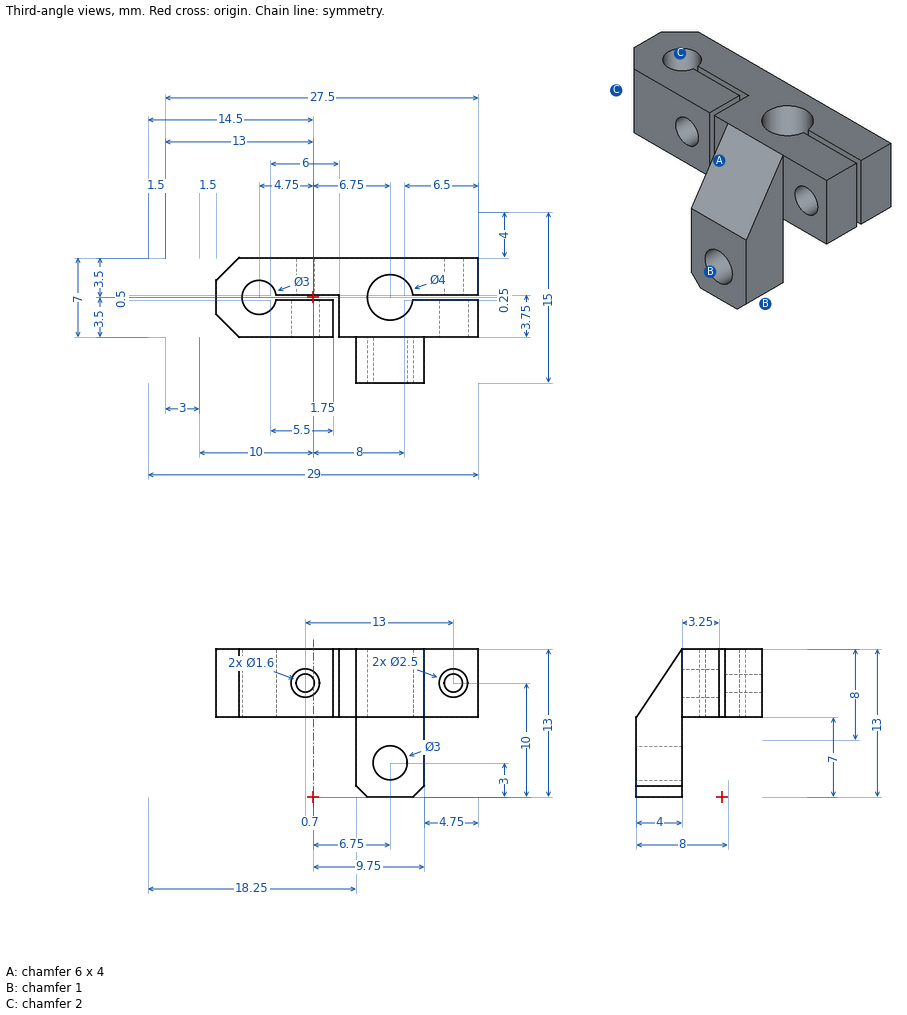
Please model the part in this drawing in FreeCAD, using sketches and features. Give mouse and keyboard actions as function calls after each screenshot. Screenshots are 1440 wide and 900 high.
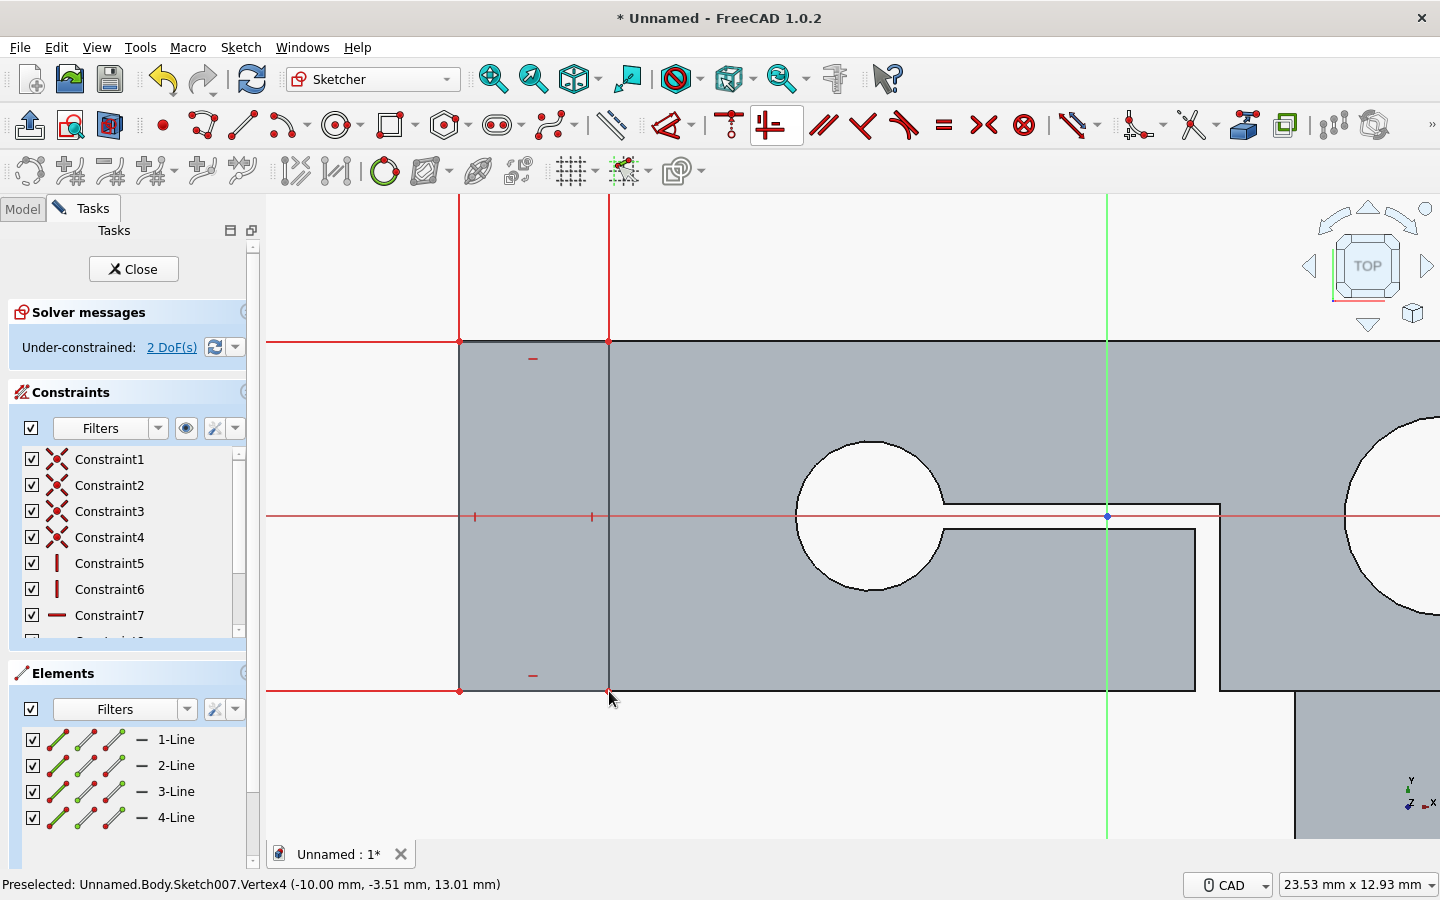
click(666, 126)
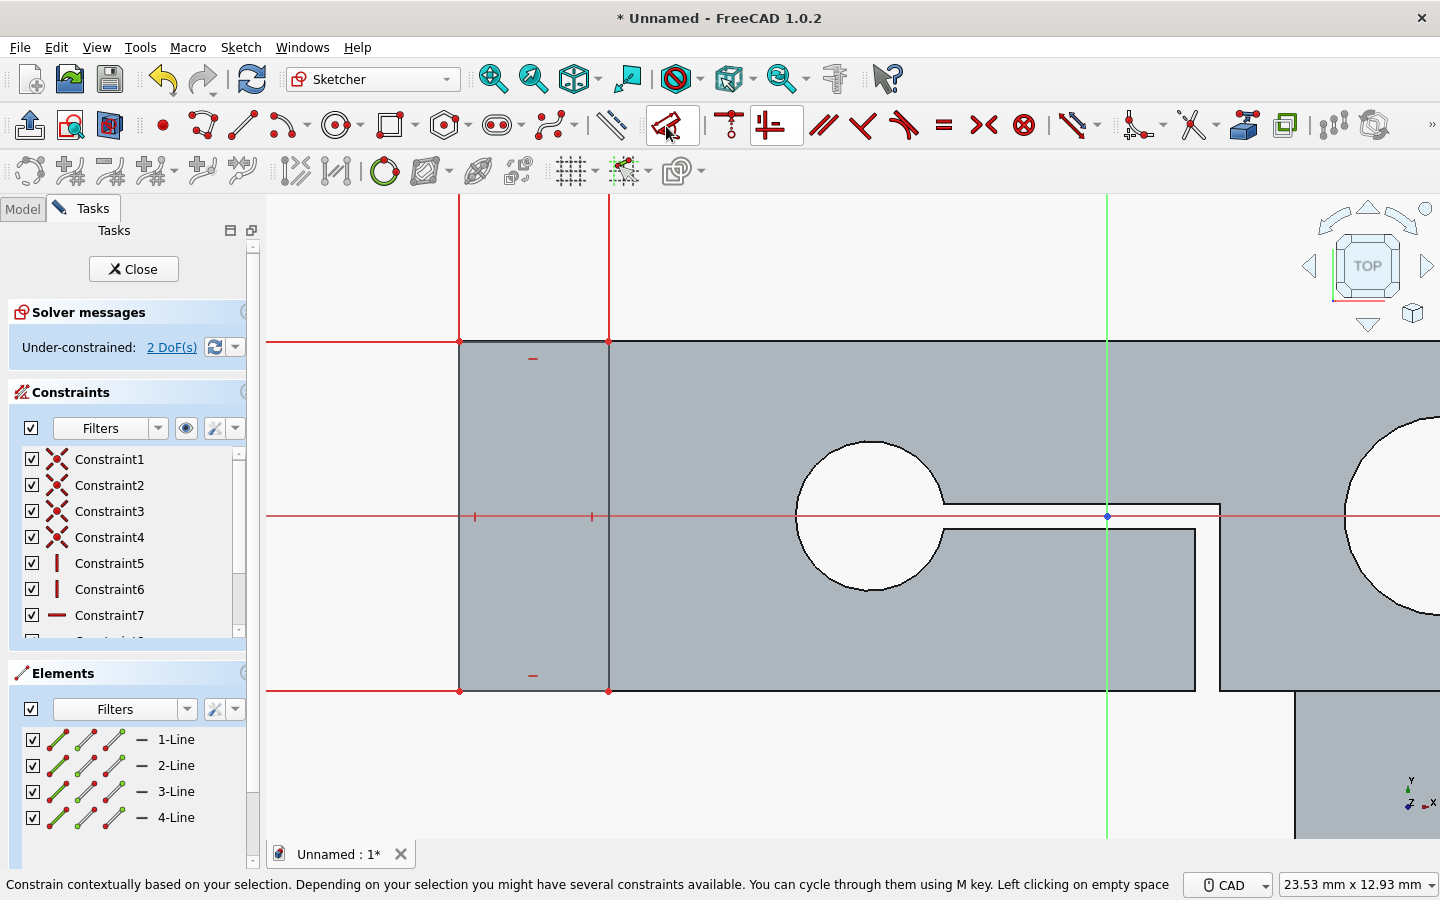
click(459, 342)
click(783, 308)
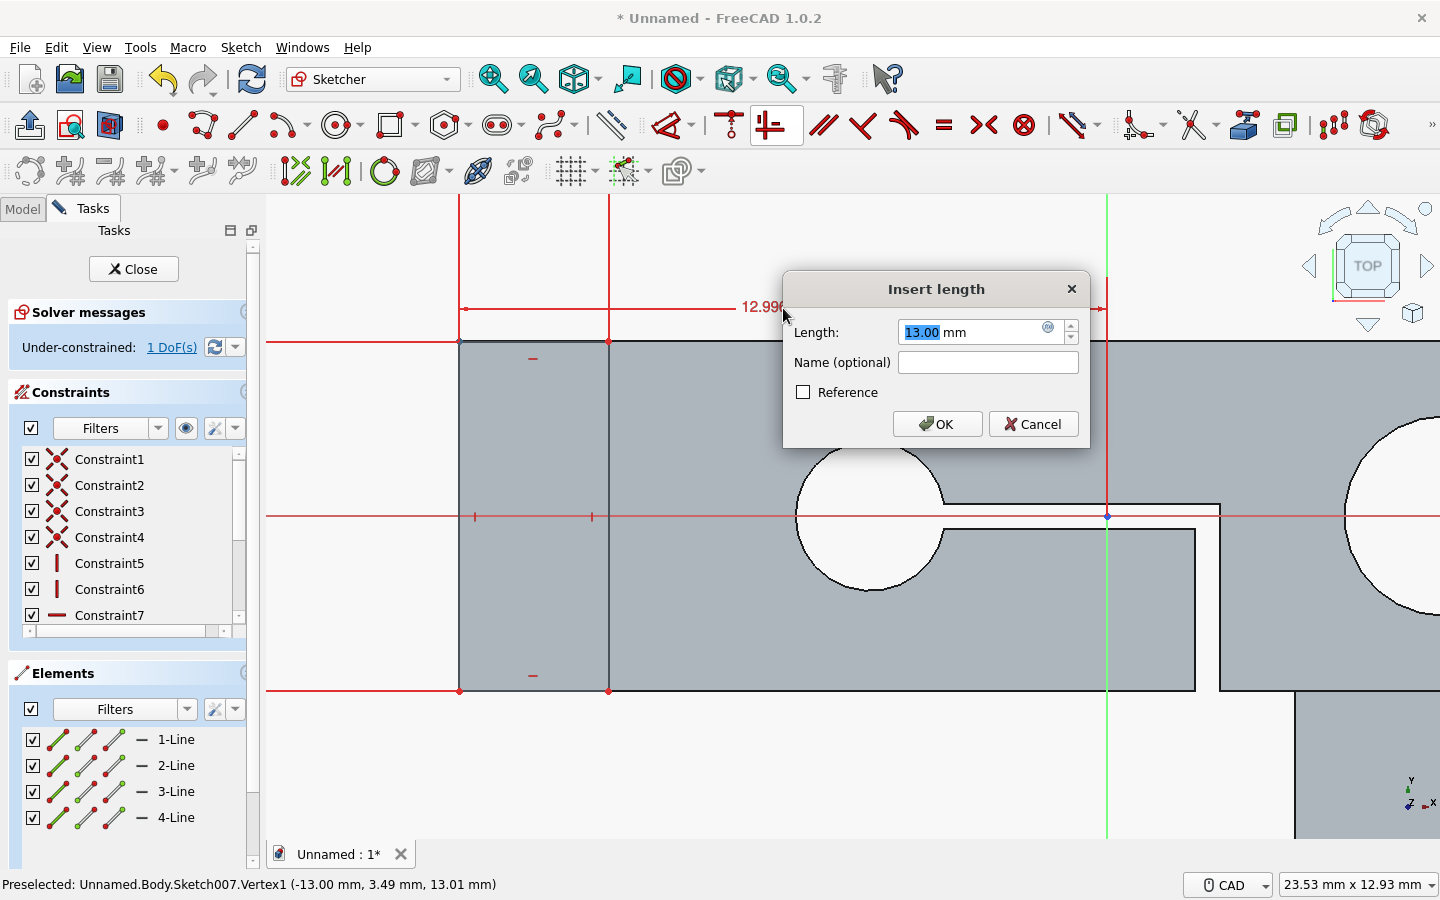
text(13)
key(Return)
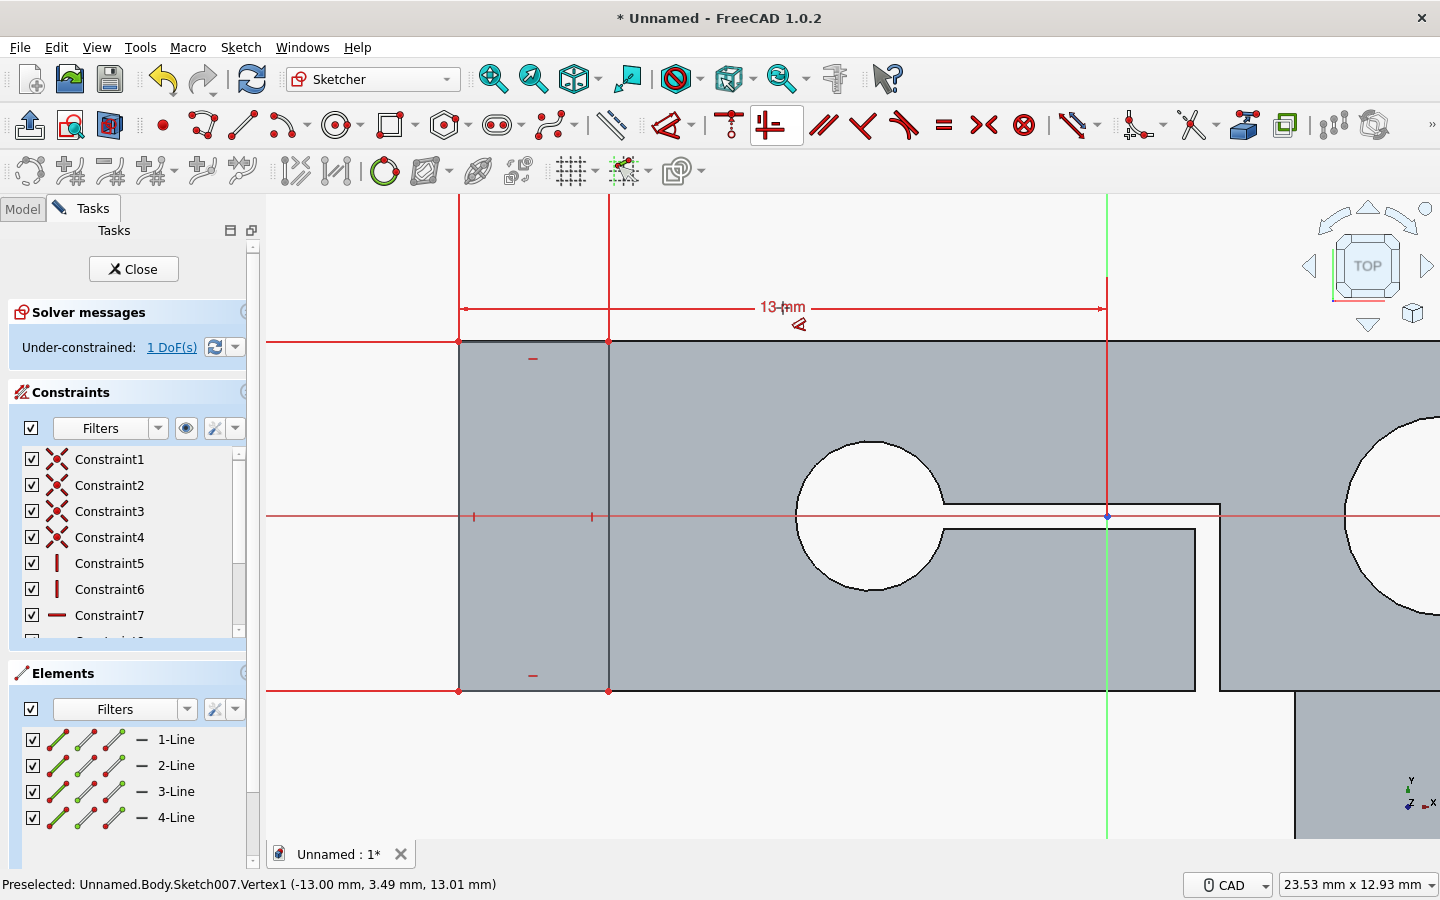
click(459, 342)
click(1141, 429)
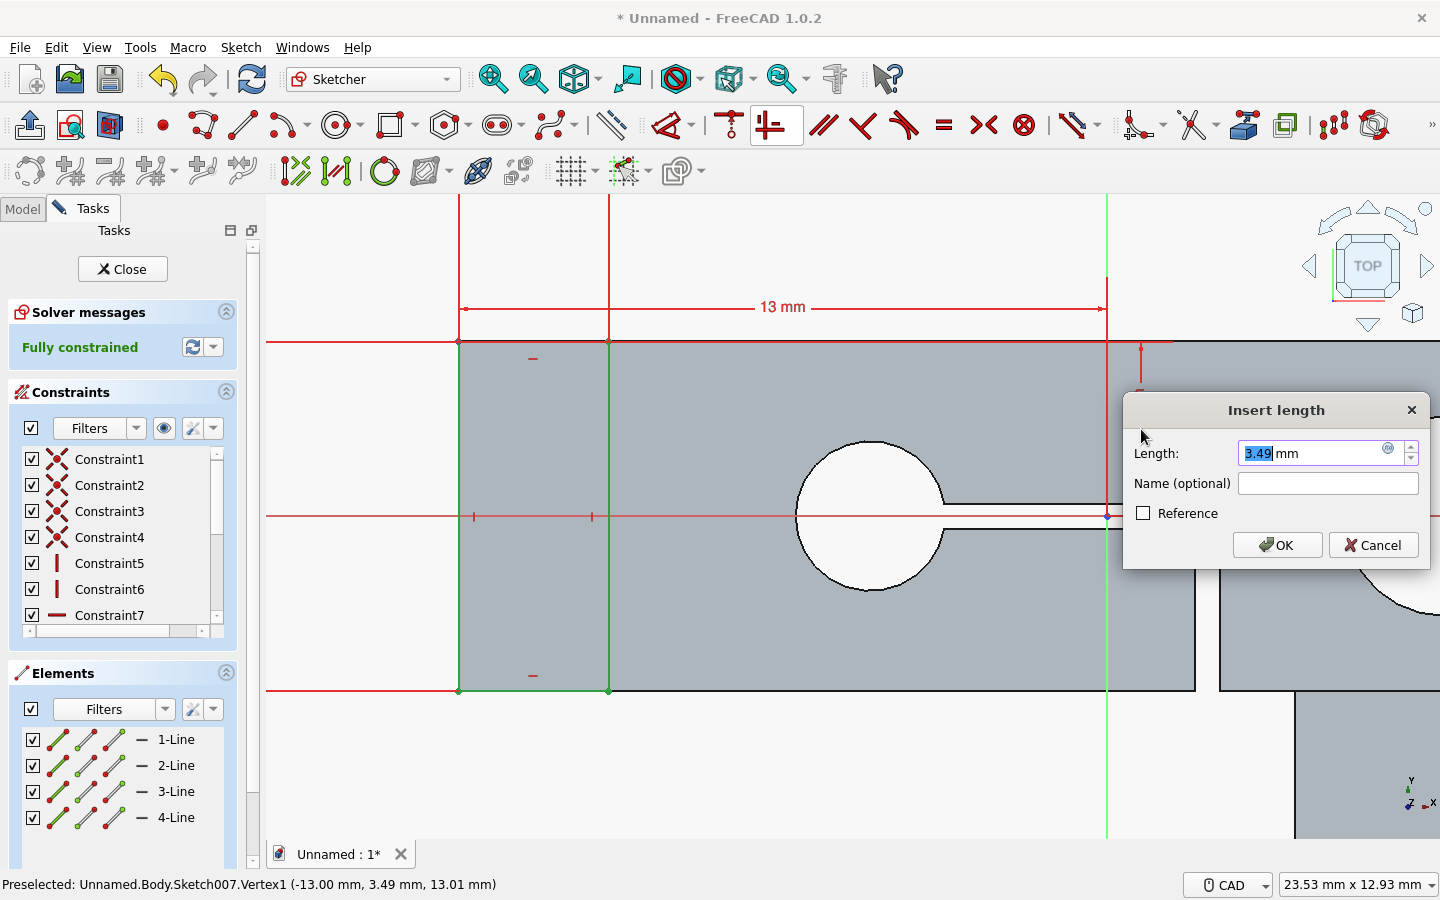
text(3.5)
key(Return)
key(Escape)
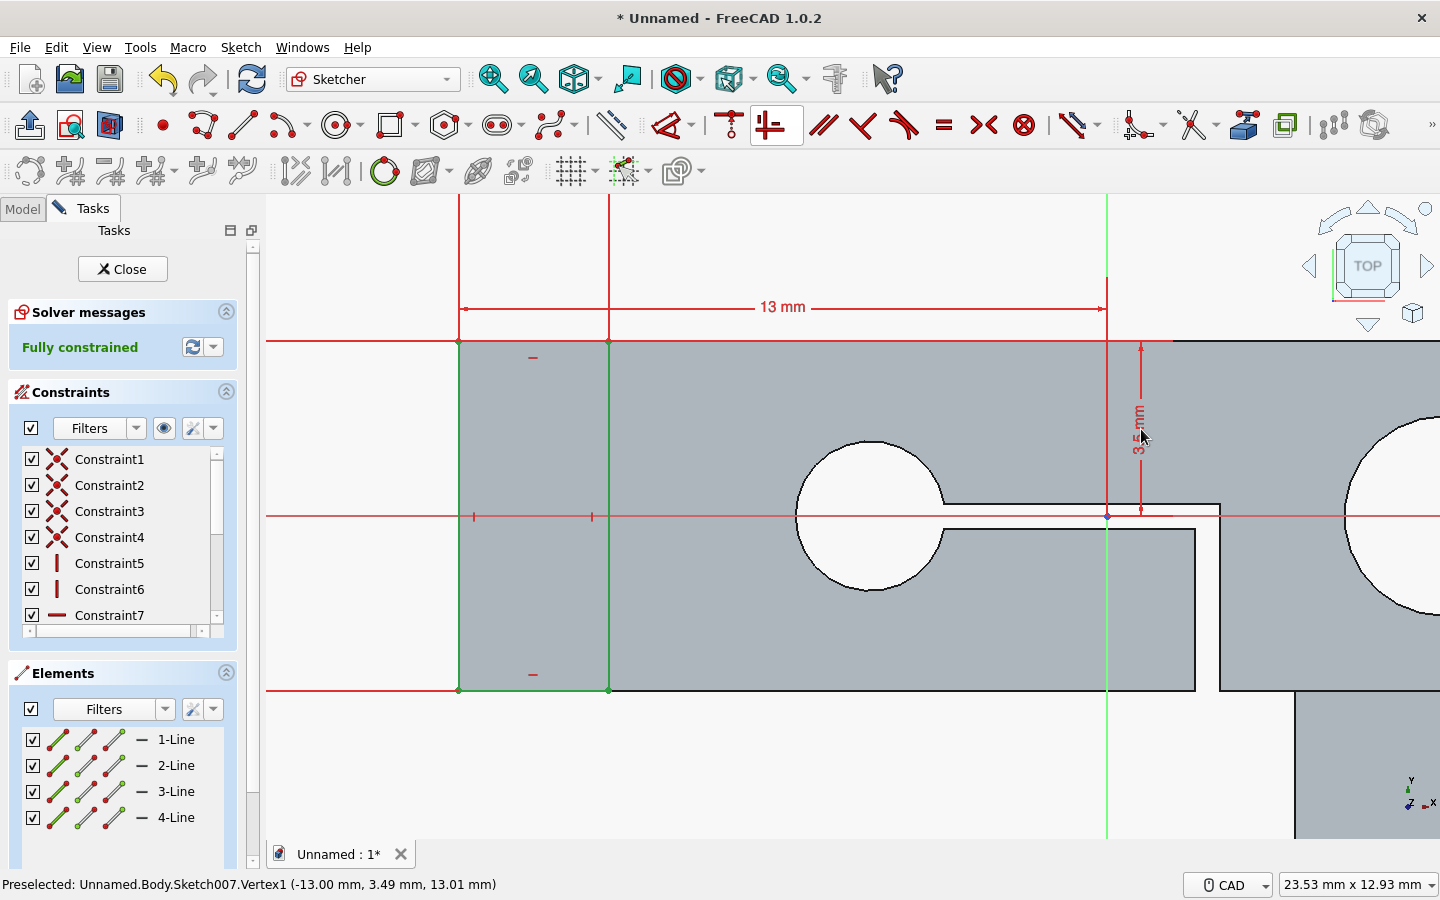
click(123, 269)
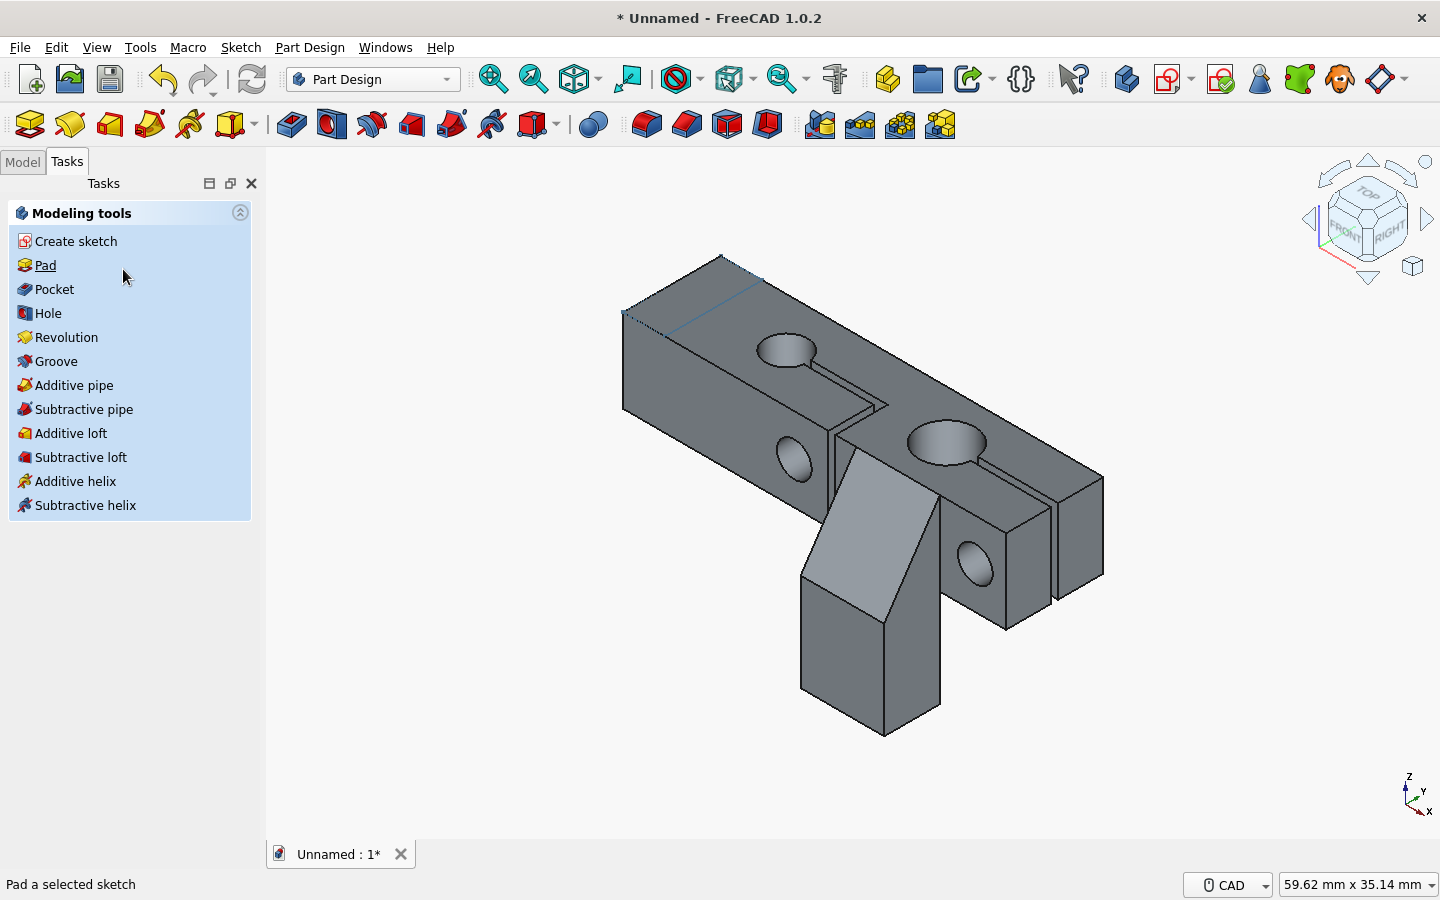
click(292, 124)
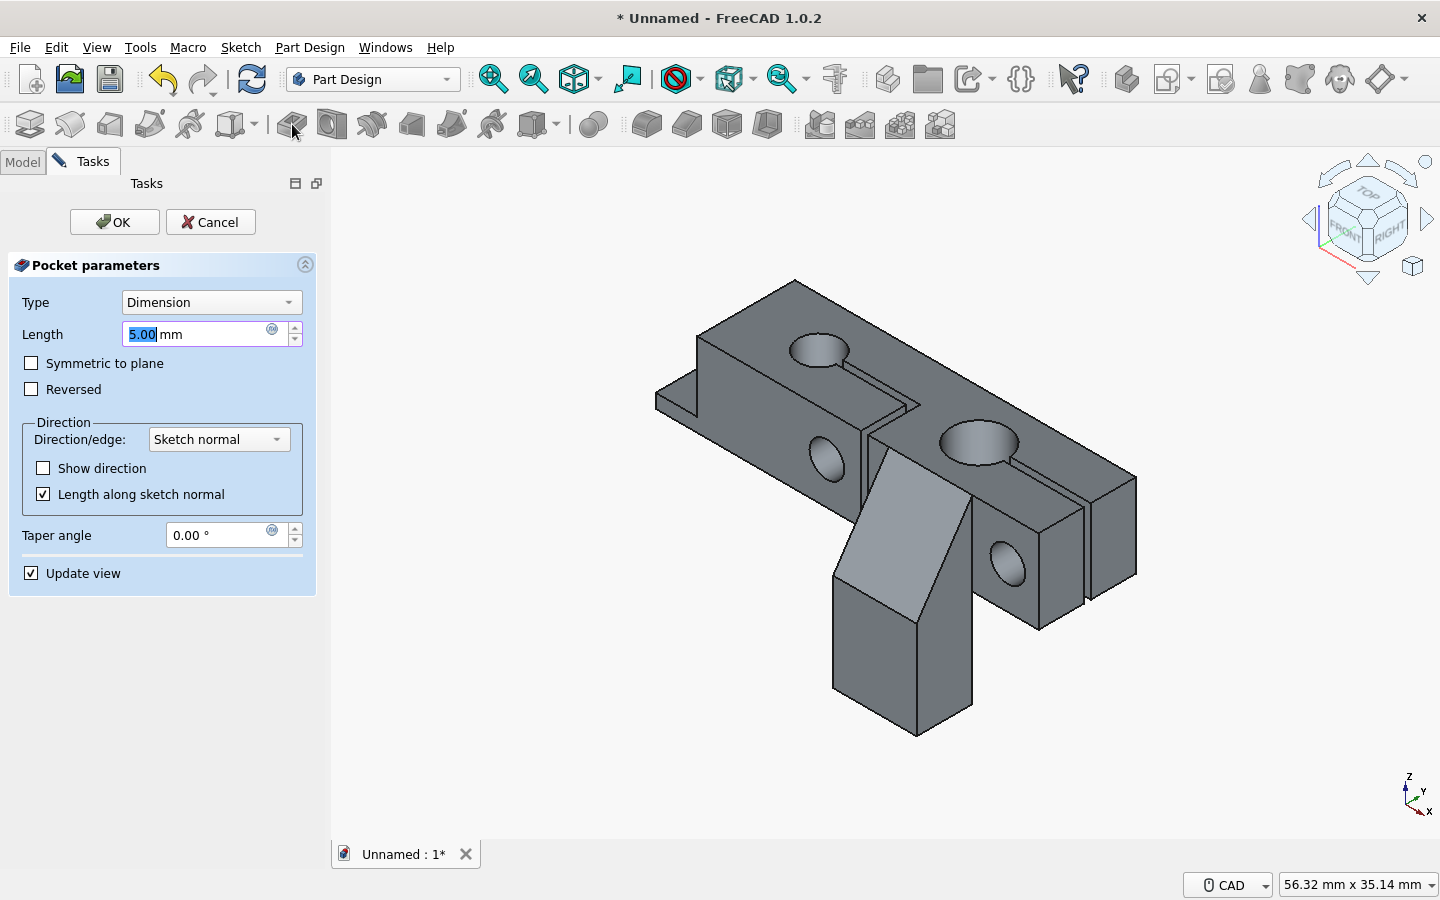
text(8)
key(Tab)